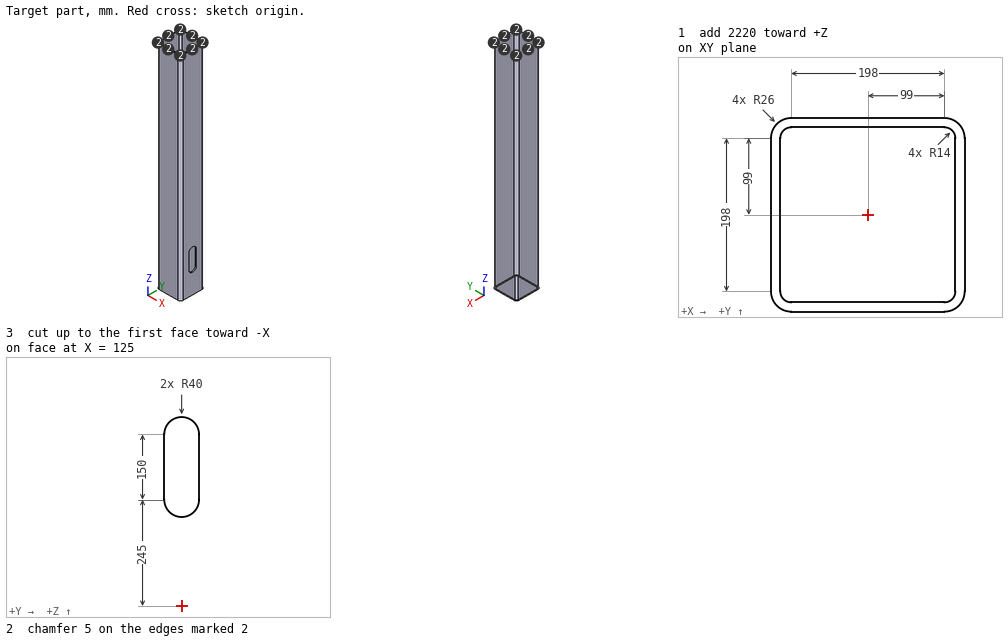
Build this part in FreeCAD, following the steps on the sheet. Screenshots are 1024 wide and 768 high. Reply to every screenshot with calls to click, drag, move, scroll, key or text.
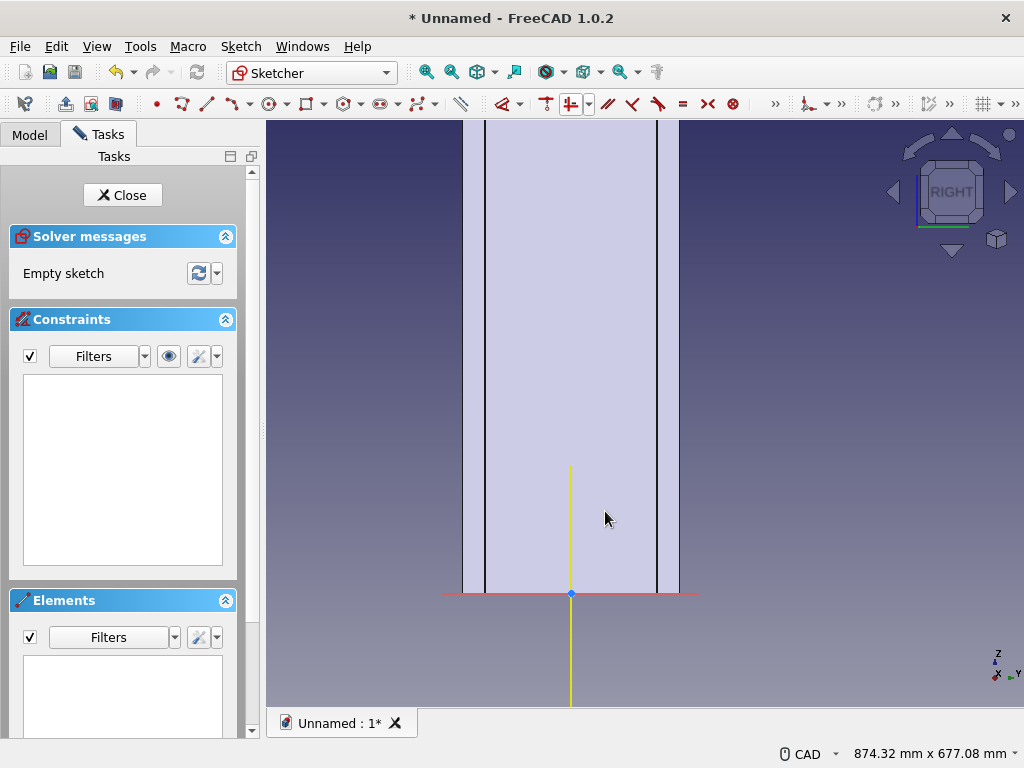
click(380, 104)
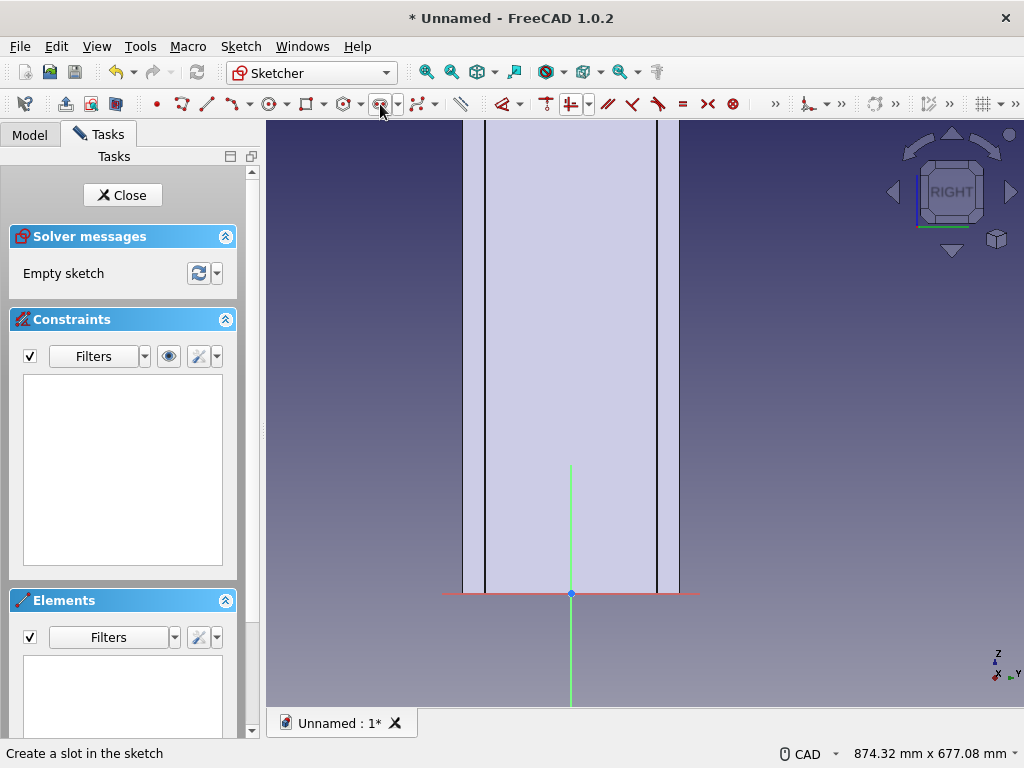
click(571, 381)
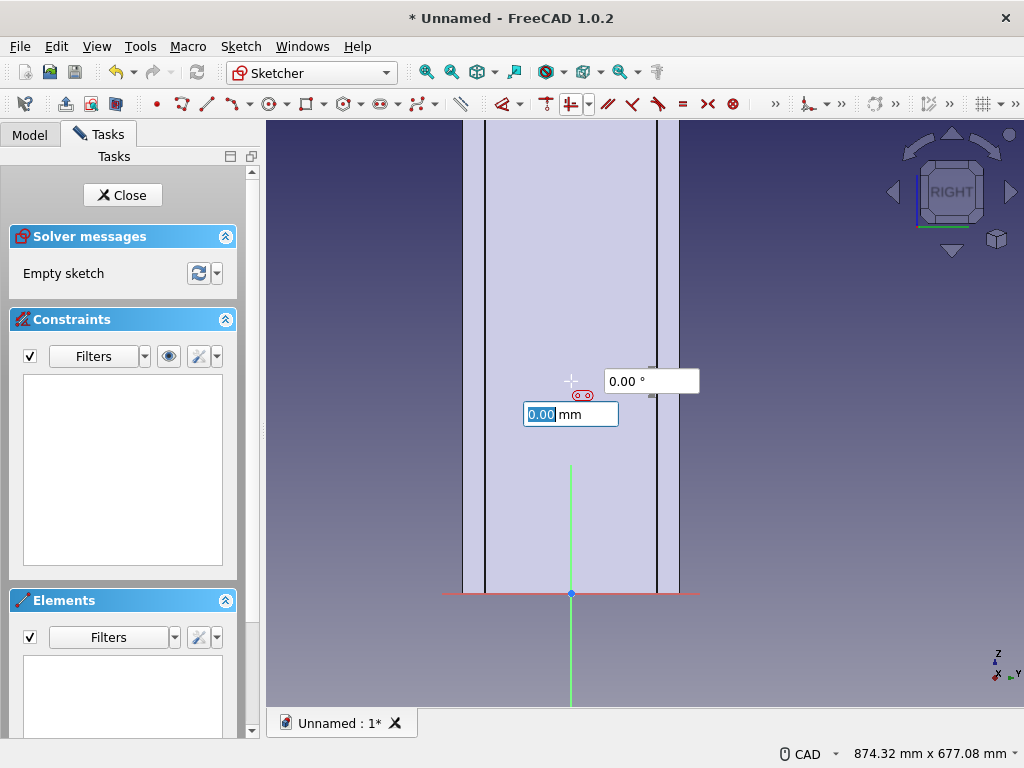
click(580, 251)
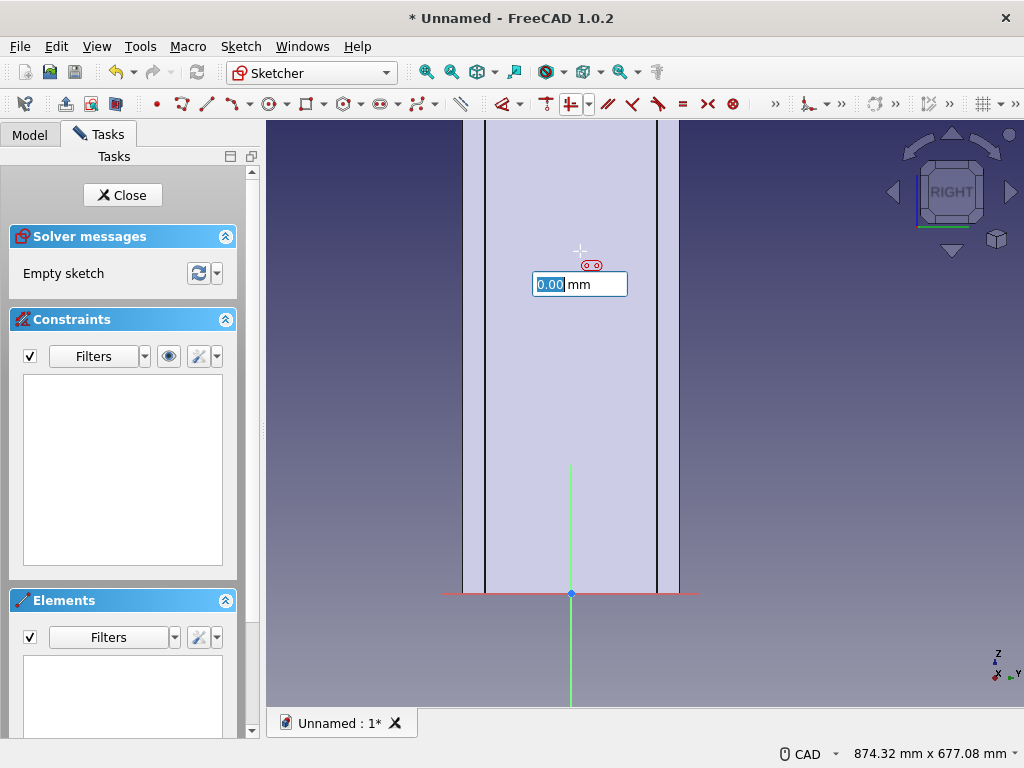
click(606, 316)
key(Escape)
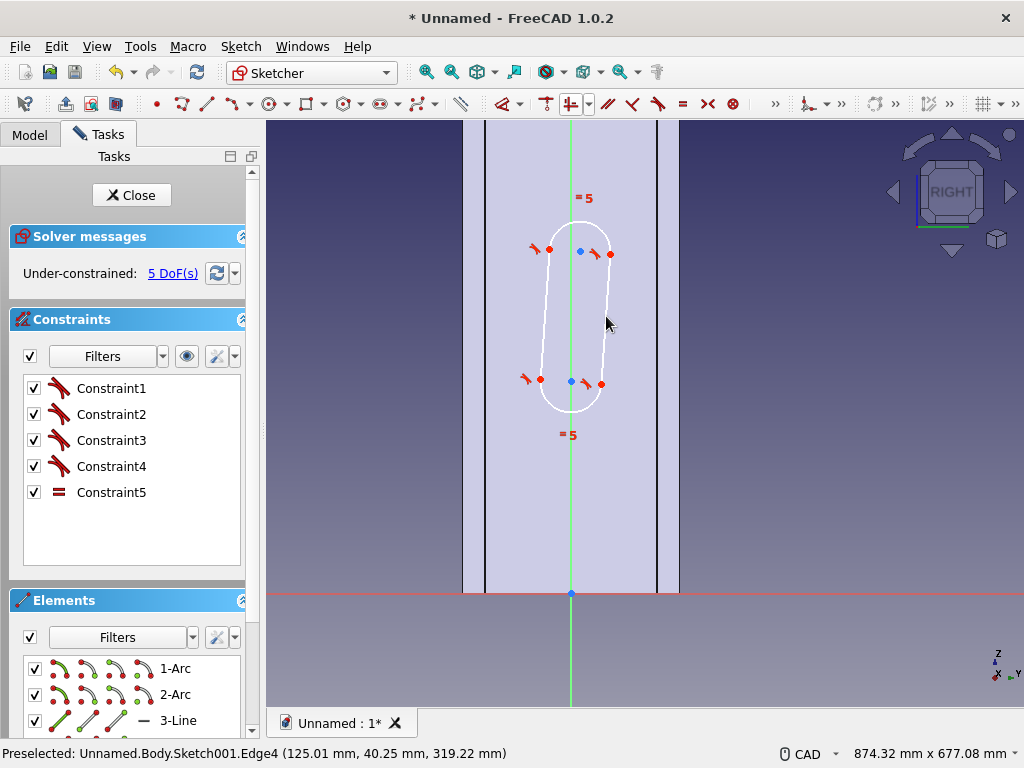
click(543, 341)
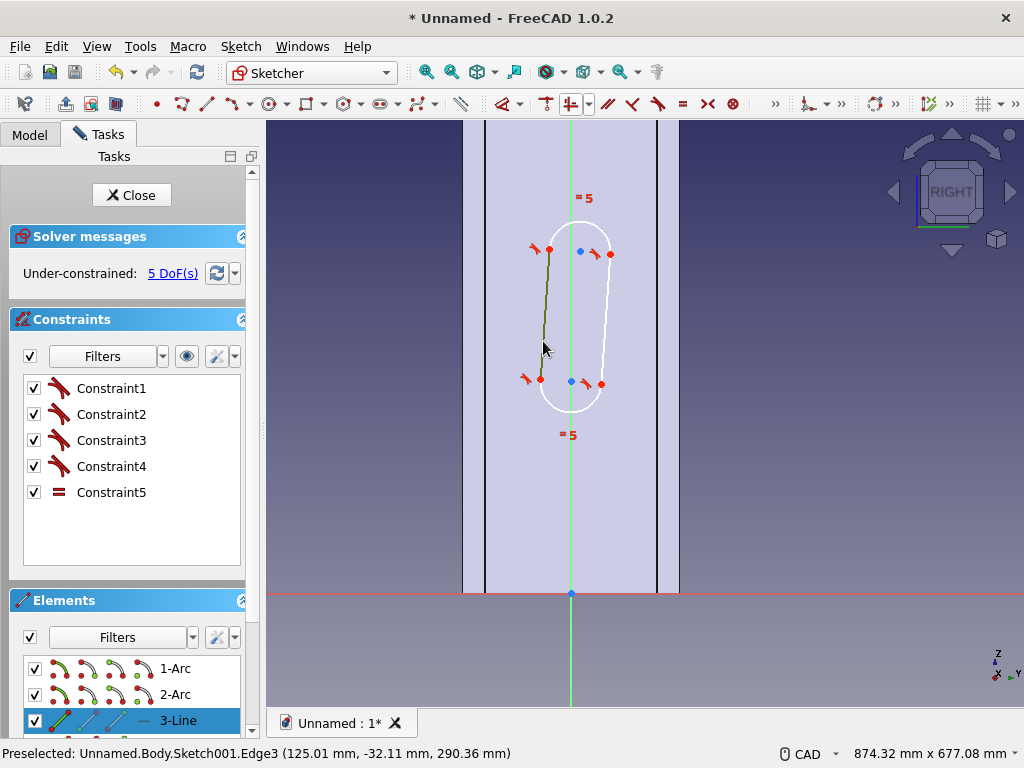
key(v)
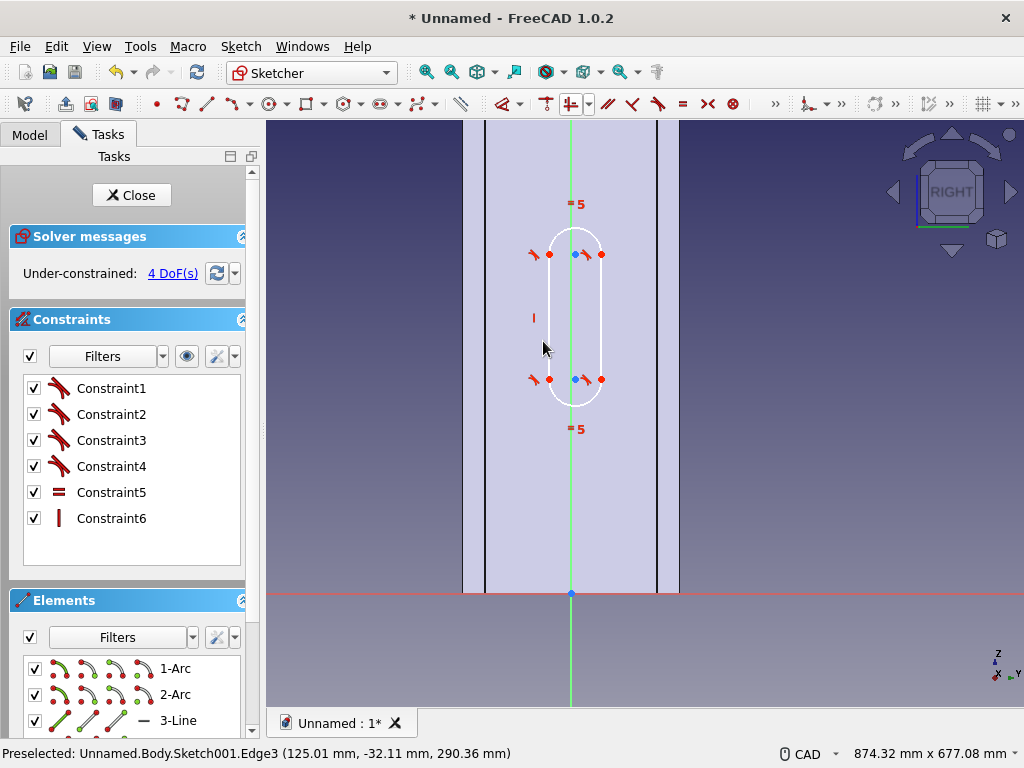
click(575, 380)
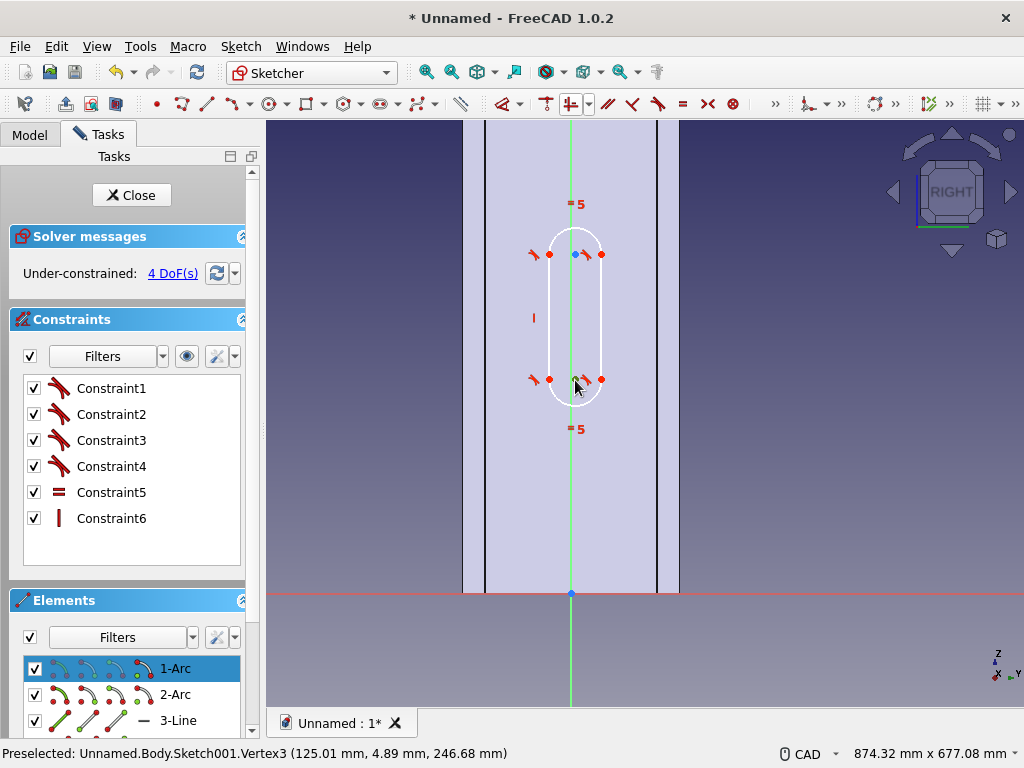
click(571, 641)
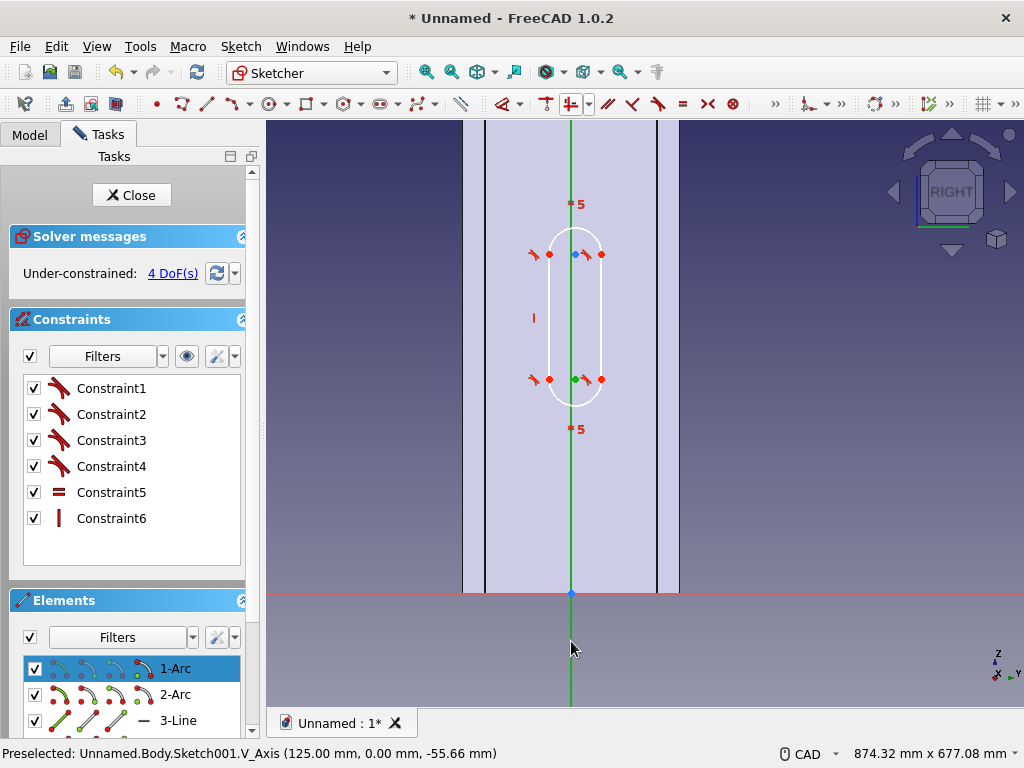
click(546, 104)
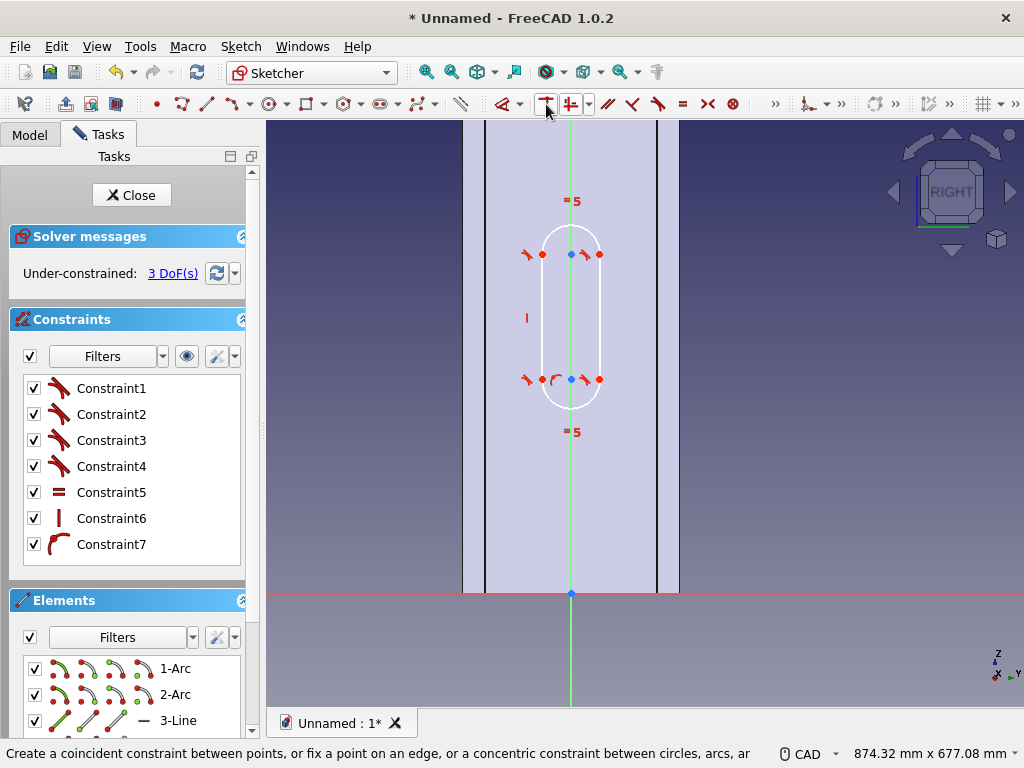
click(502, 104)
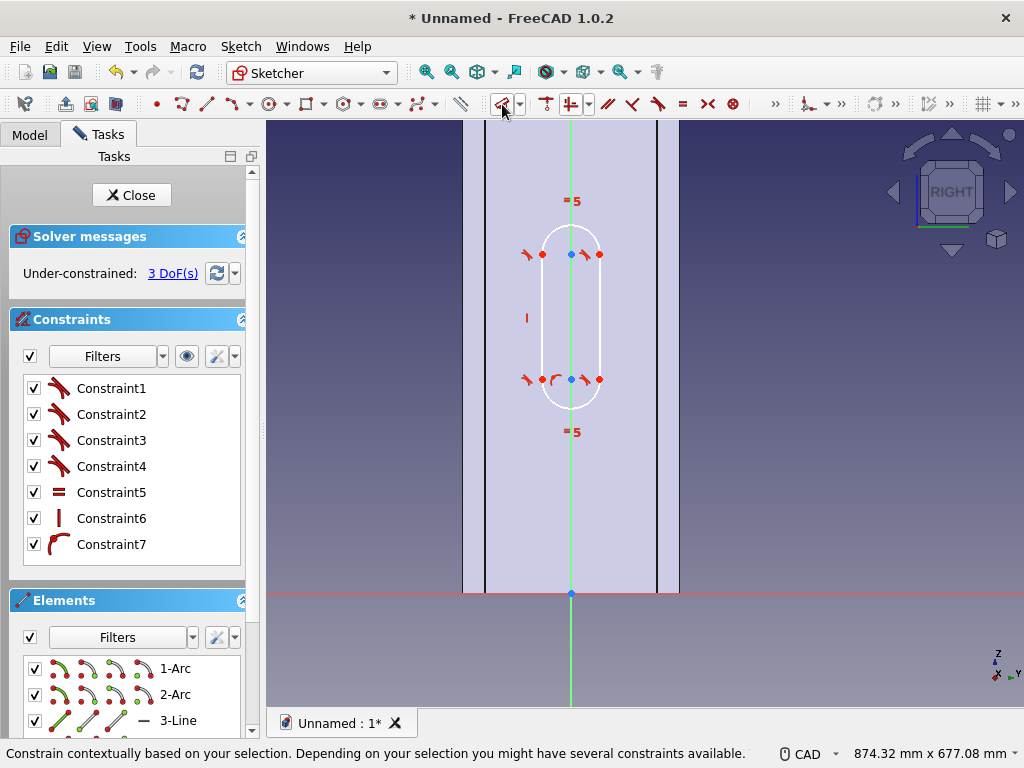
click(554, 403)
click(535, 429)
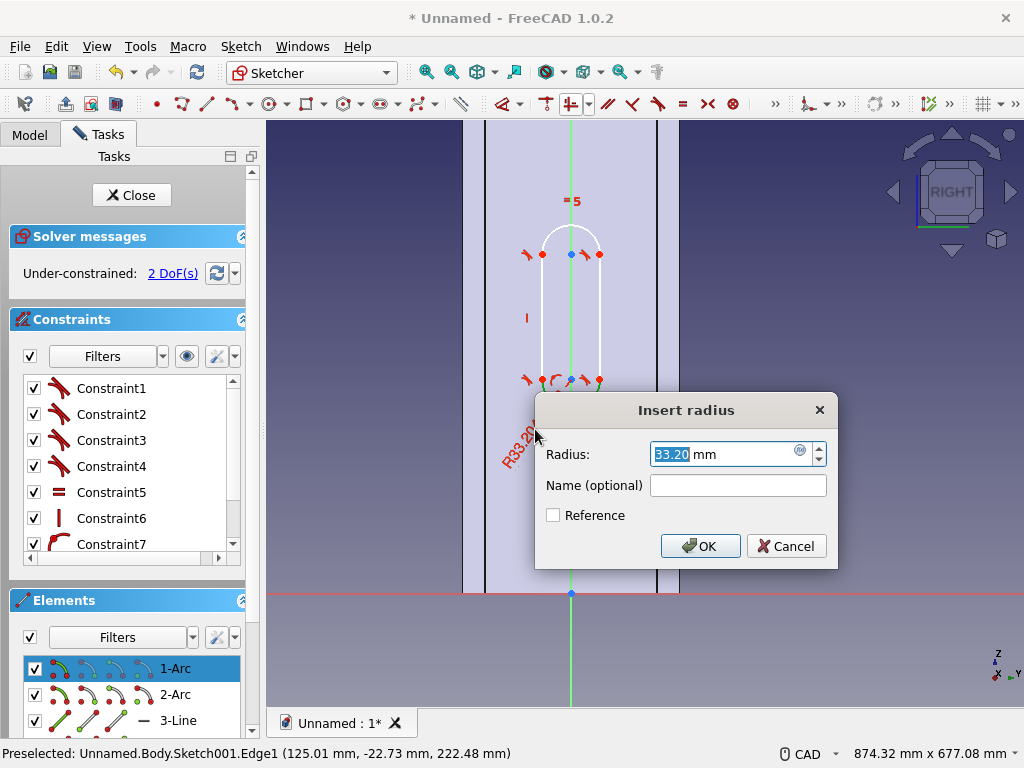
text(40)
key(Return)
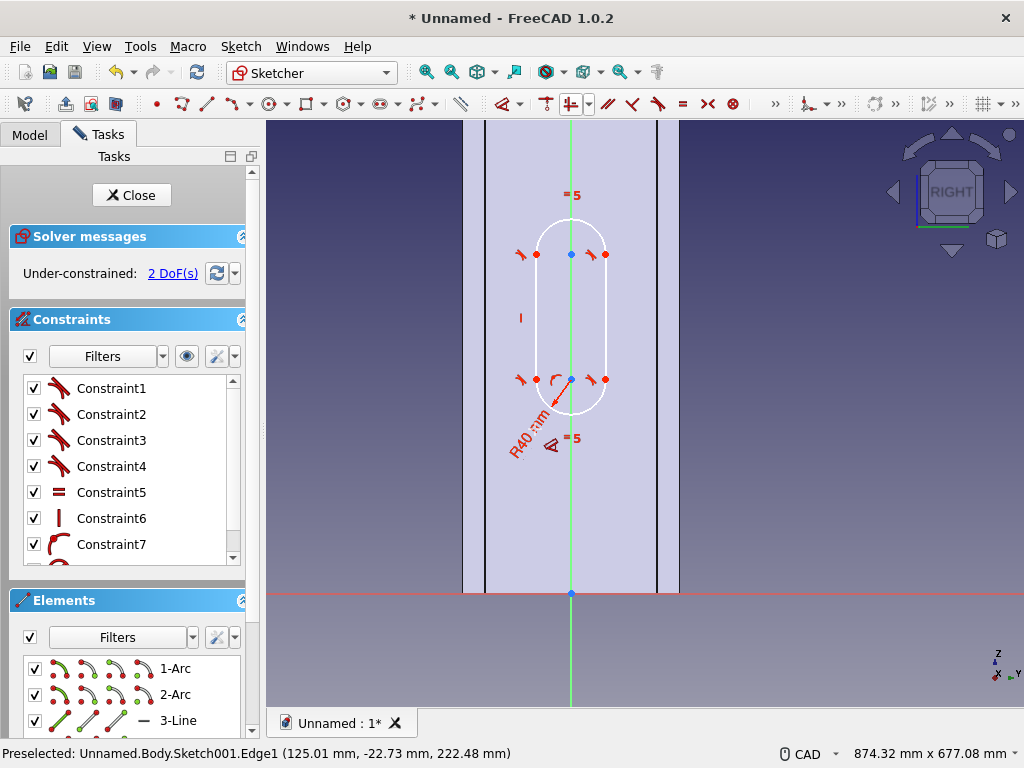
click(536, 342)
click(502, 317)